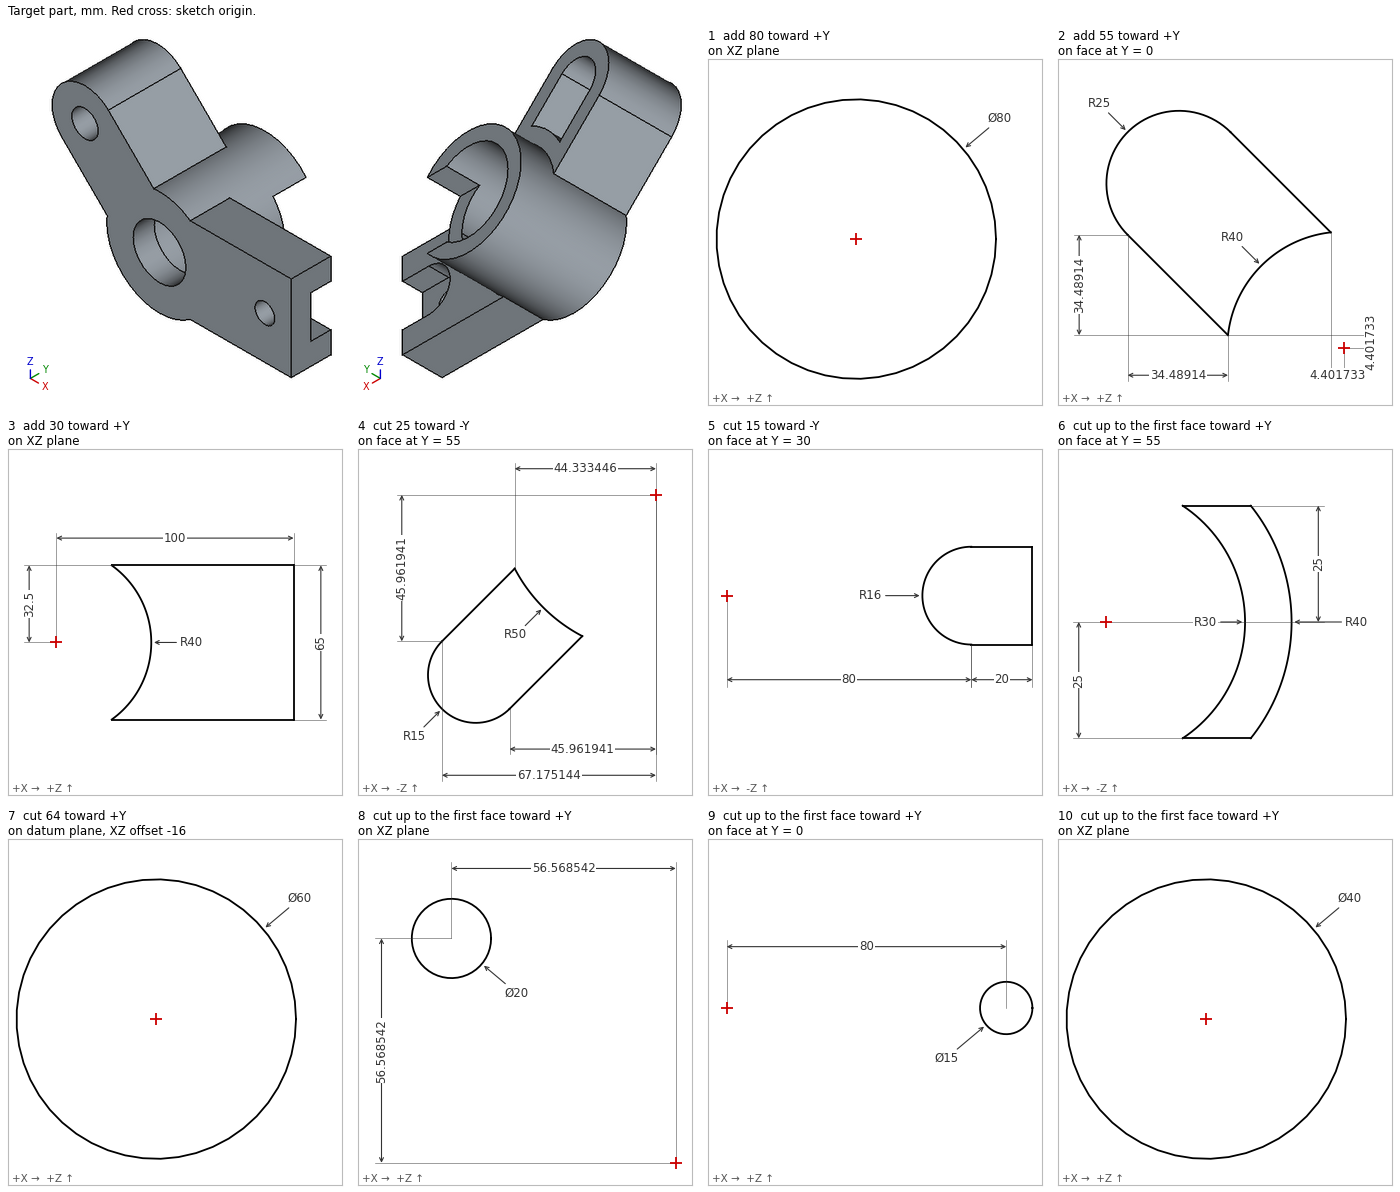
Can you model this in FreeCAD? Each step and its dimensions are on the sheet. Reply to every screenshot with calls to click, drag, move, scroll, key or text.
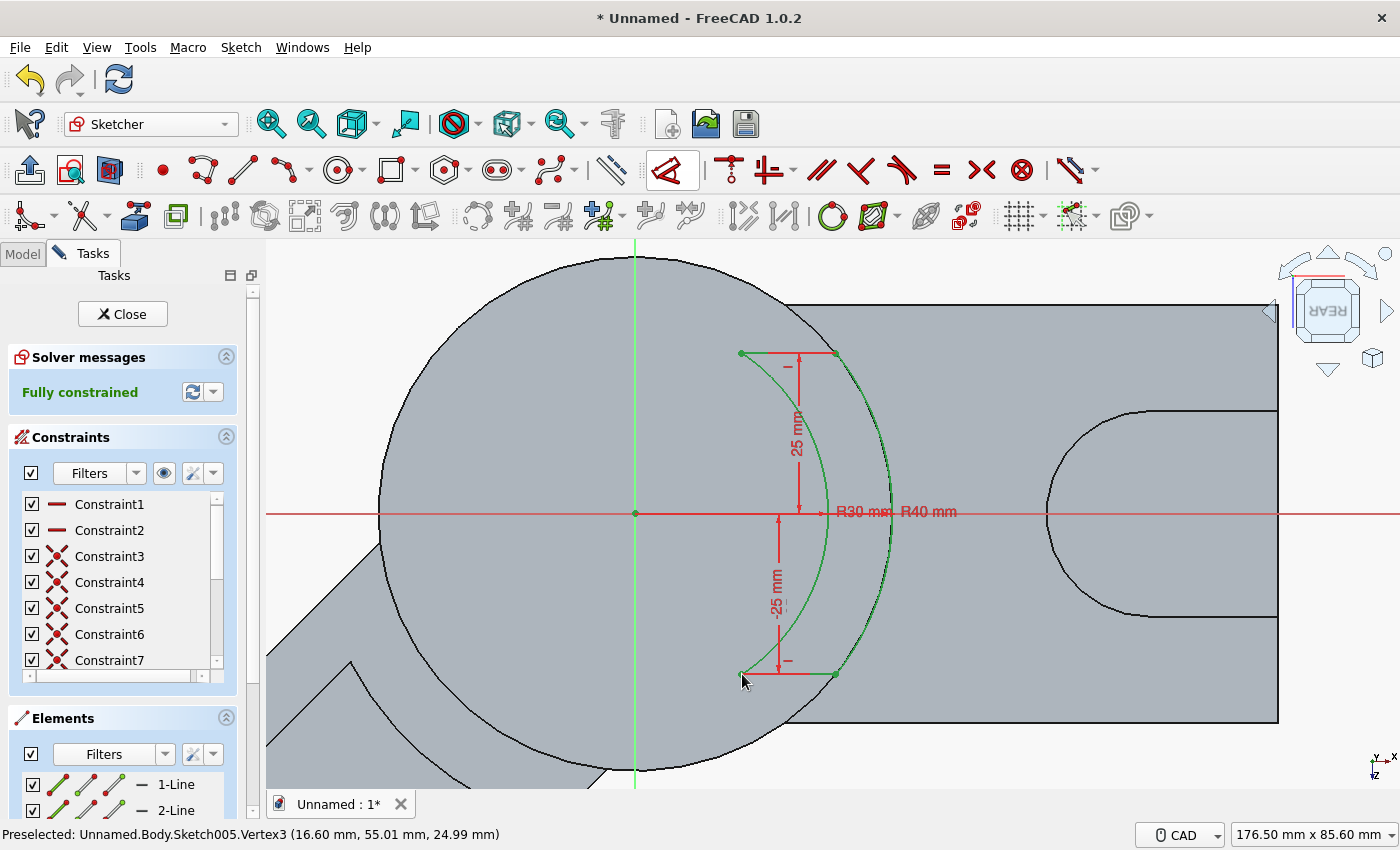
click(123, 314)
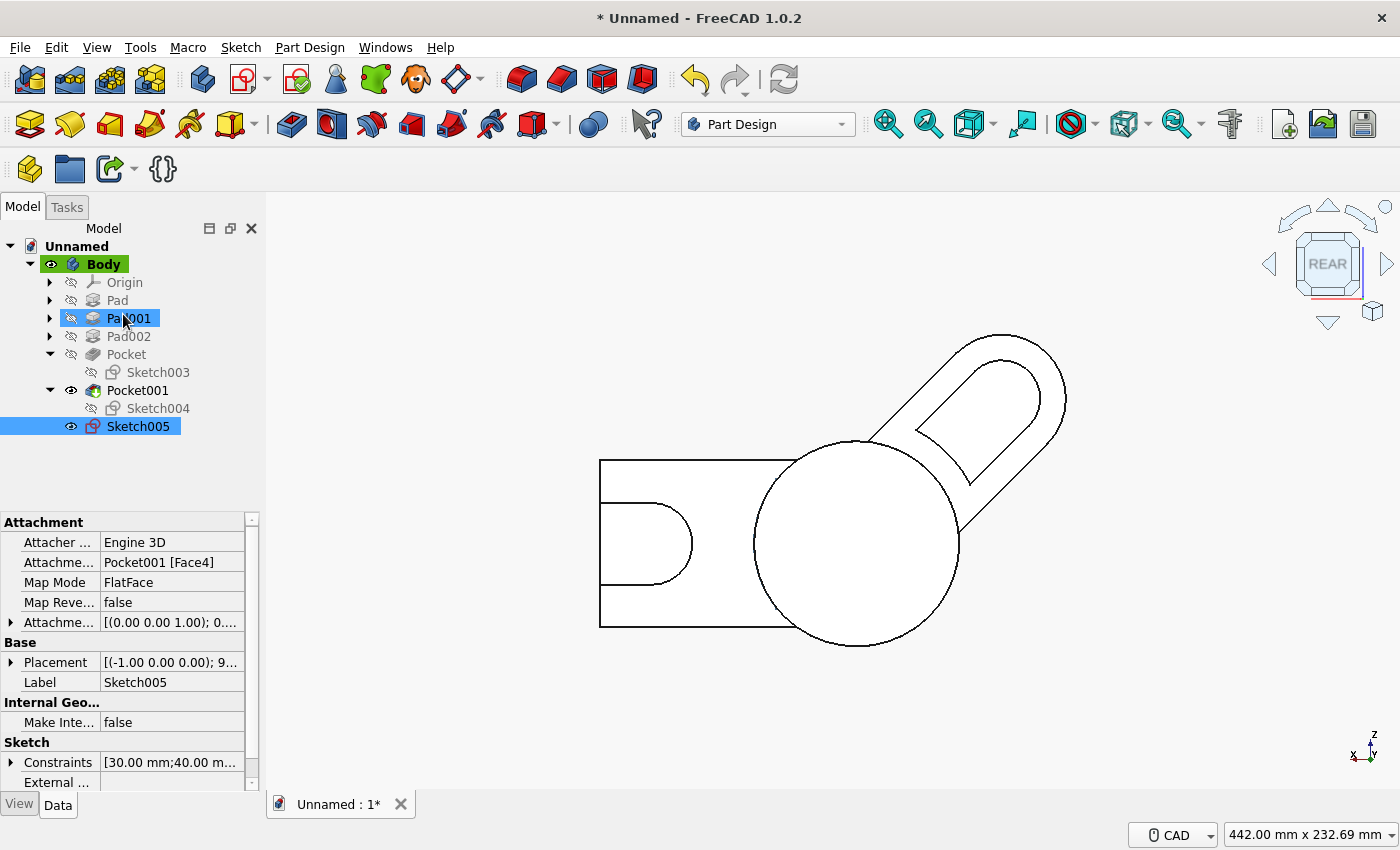
click(292, 124)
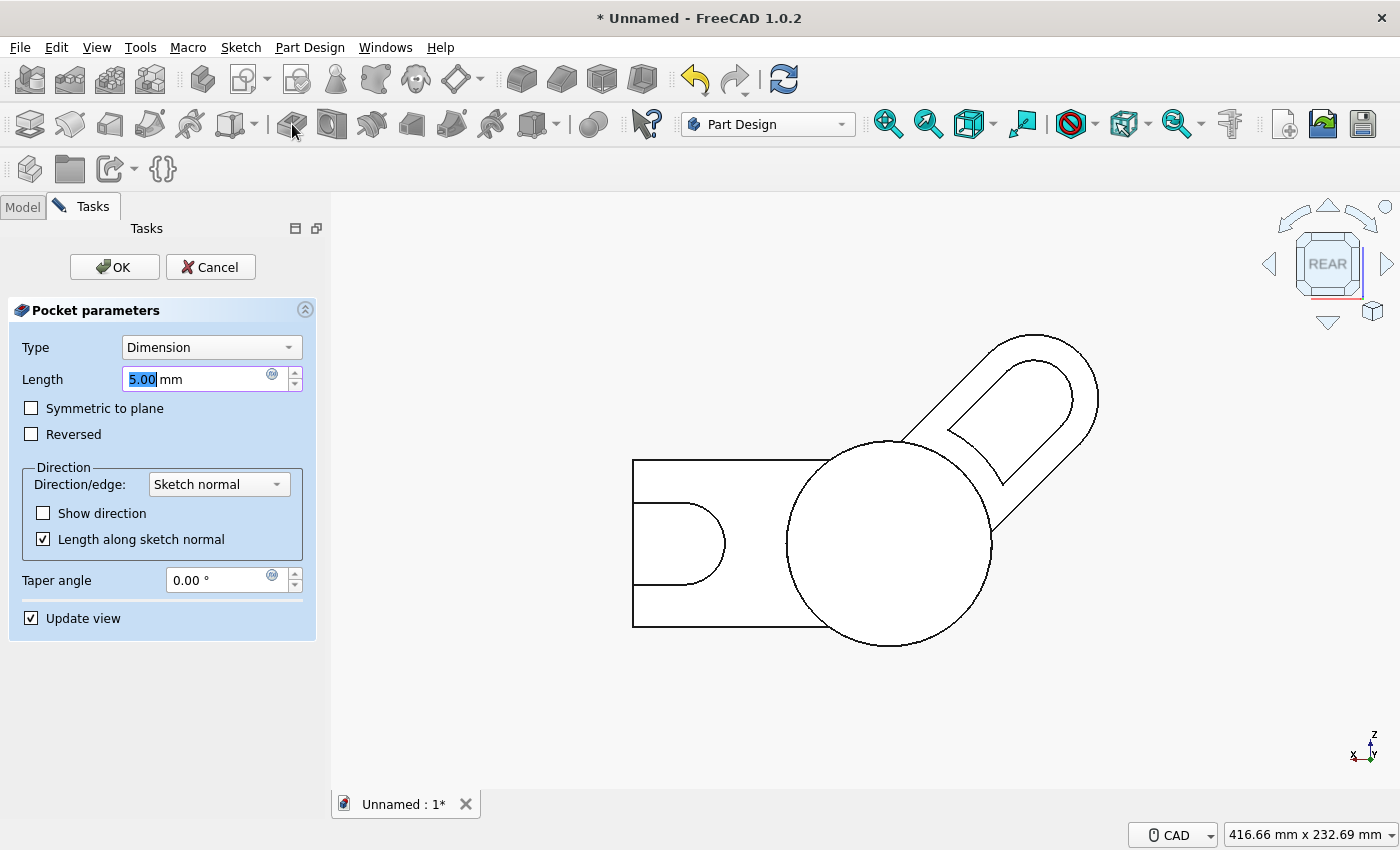
click(212, 348)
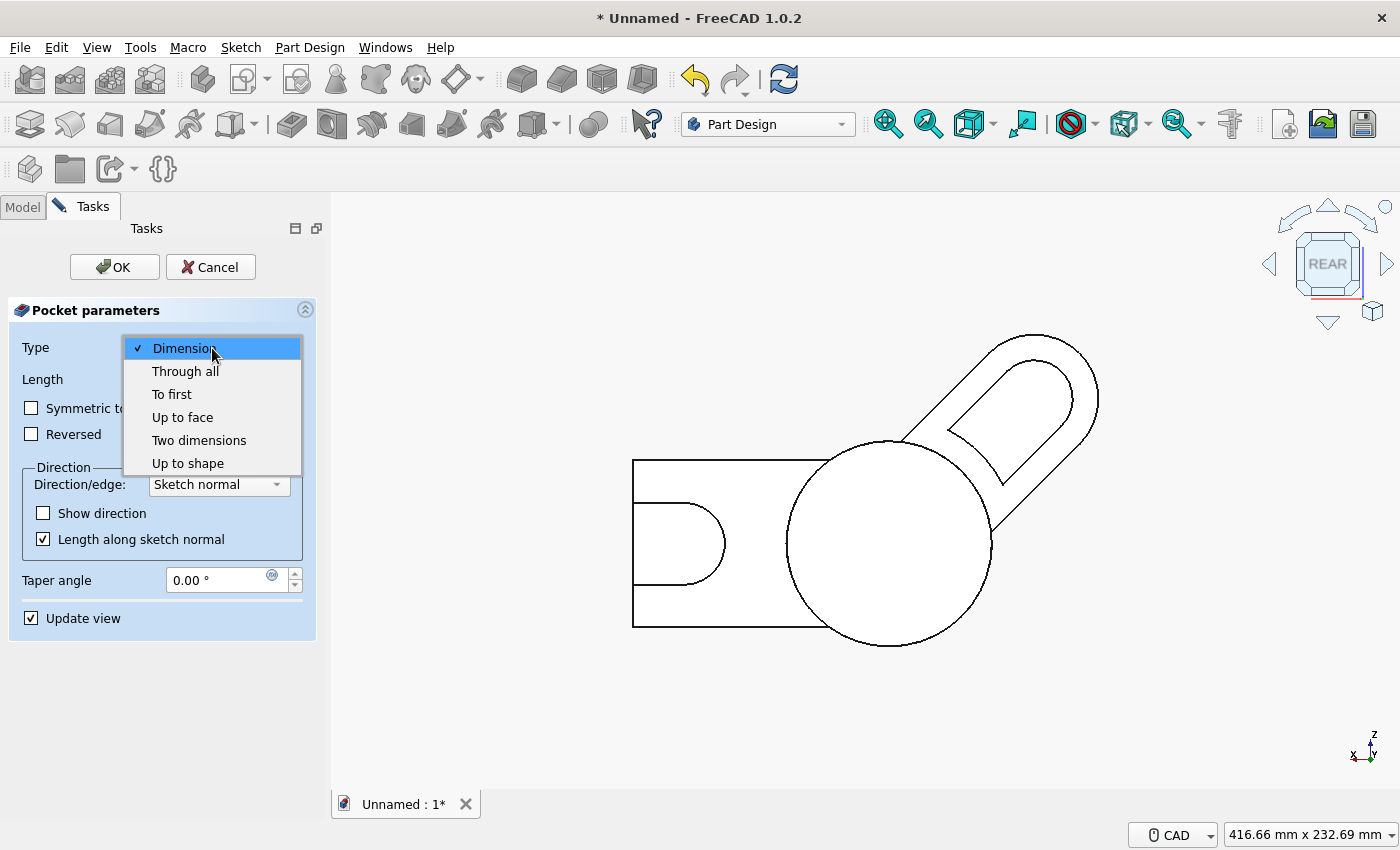
click(212, 394)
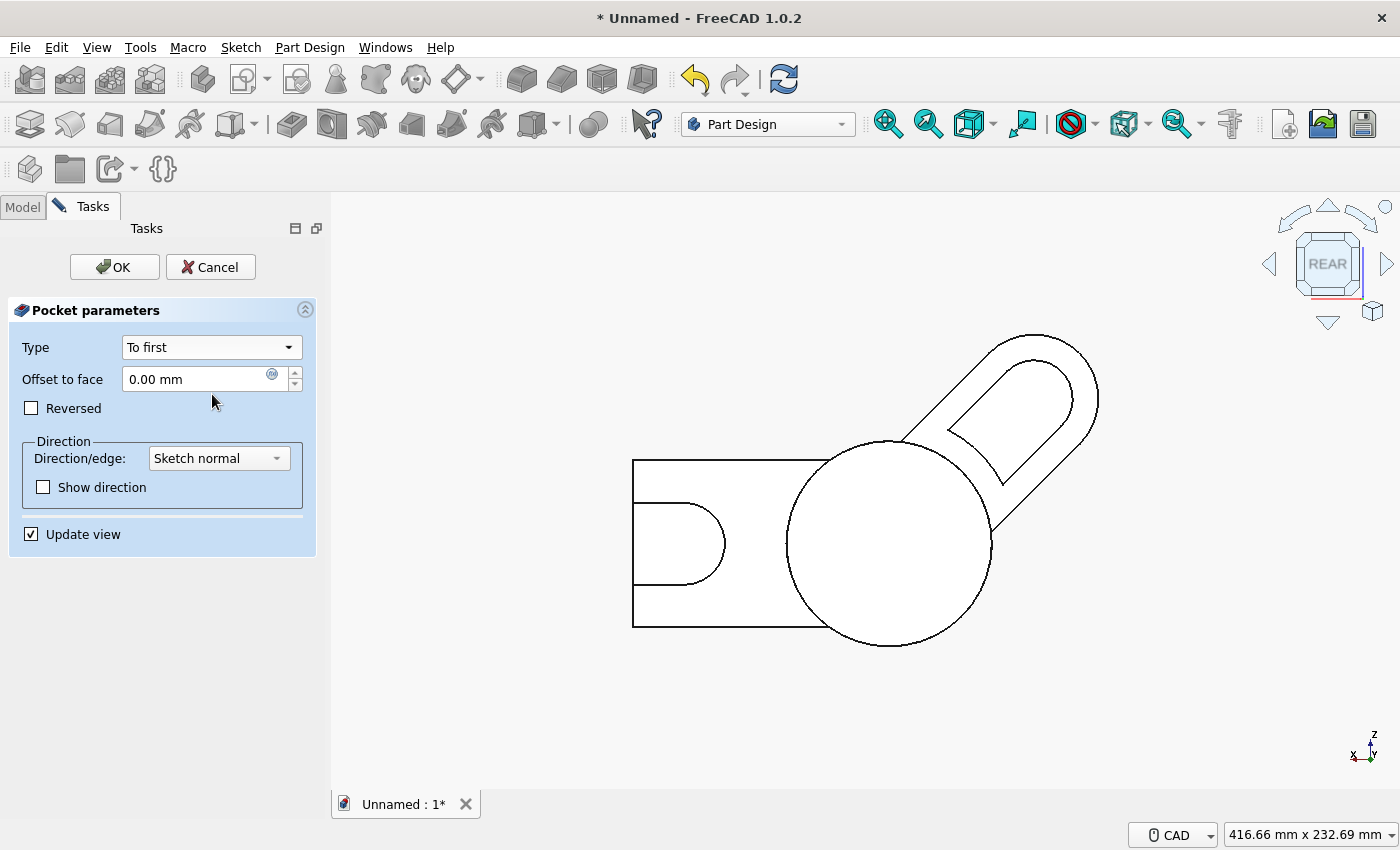
click(30, 408)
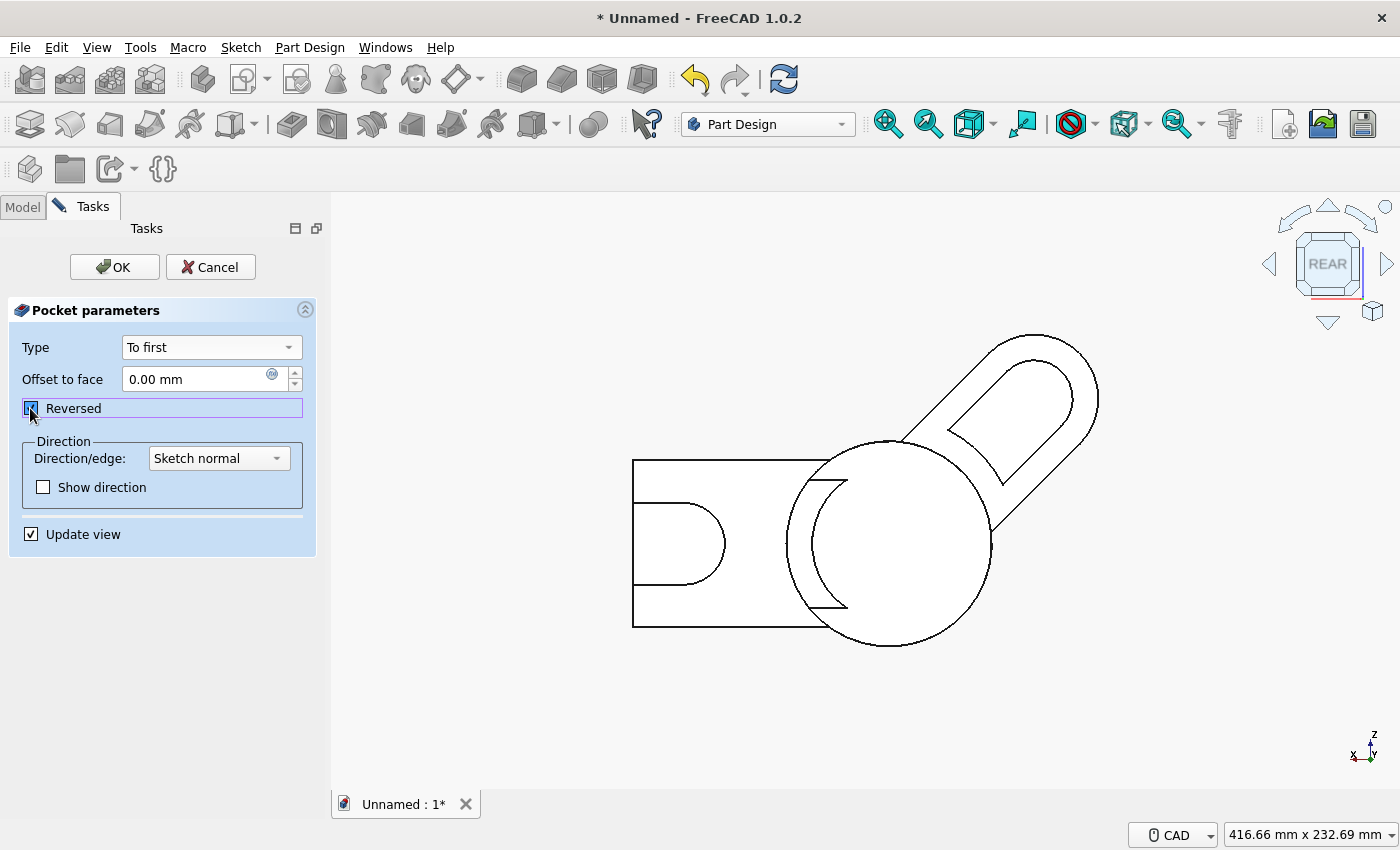
click(115, 267)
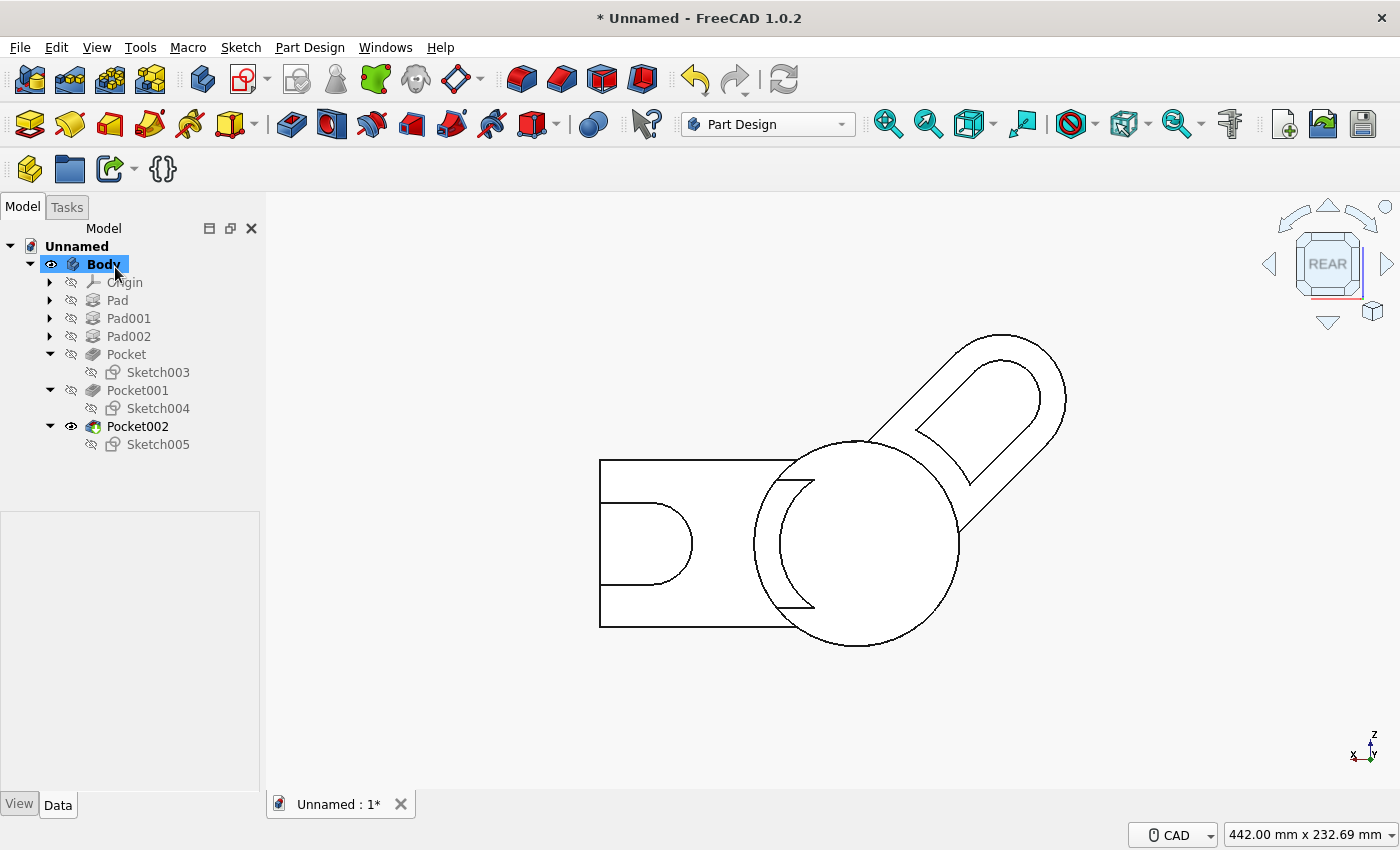
click(50, 282)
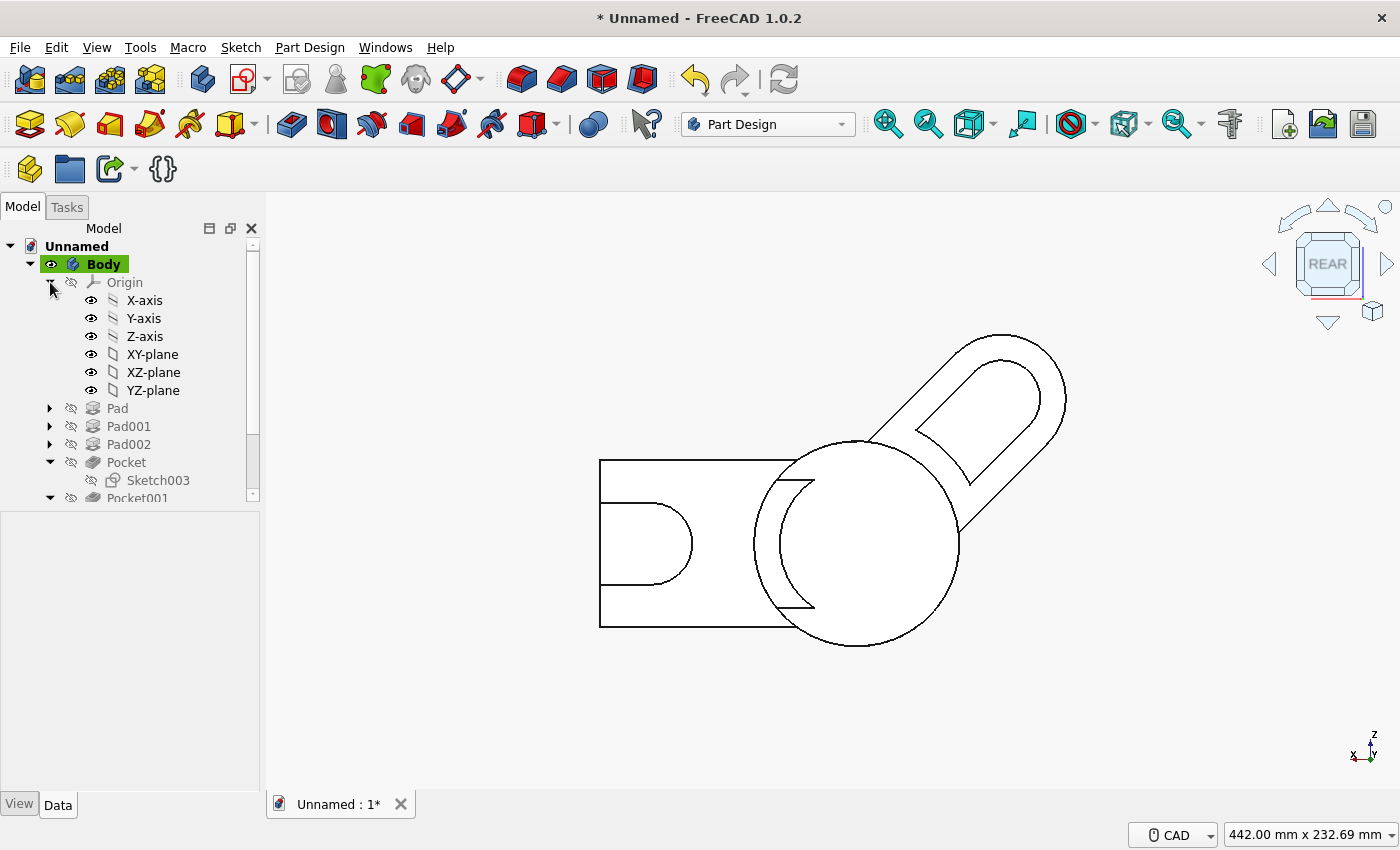
click(136, 372)